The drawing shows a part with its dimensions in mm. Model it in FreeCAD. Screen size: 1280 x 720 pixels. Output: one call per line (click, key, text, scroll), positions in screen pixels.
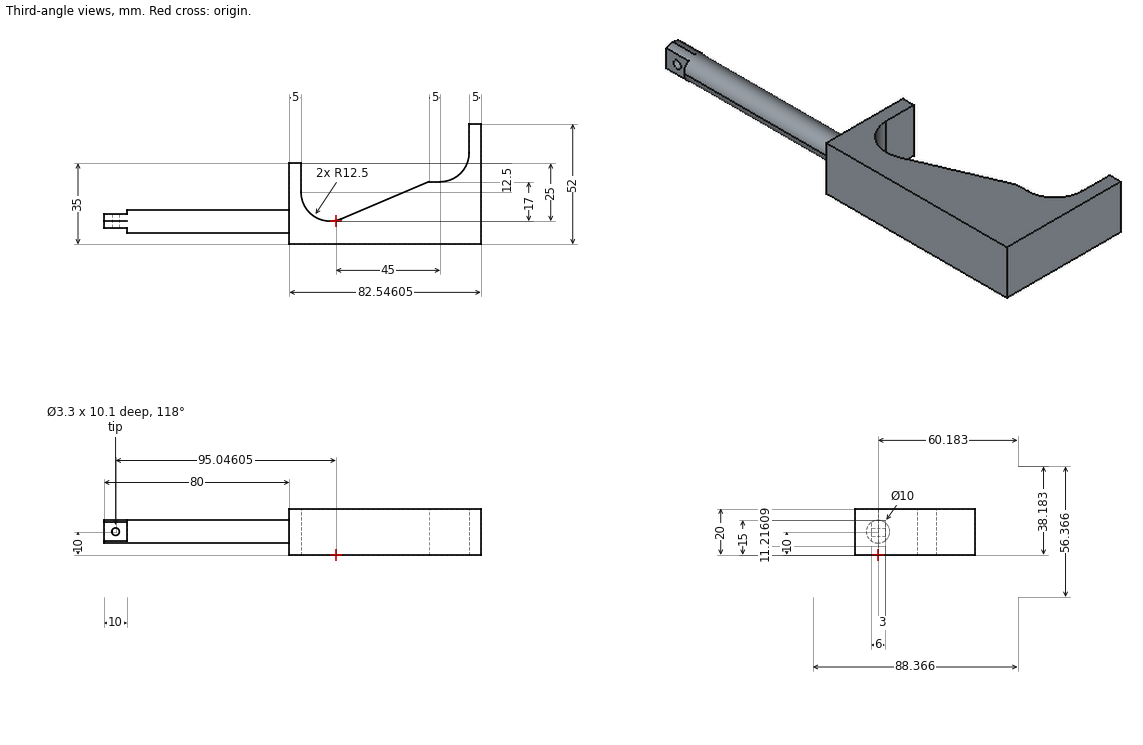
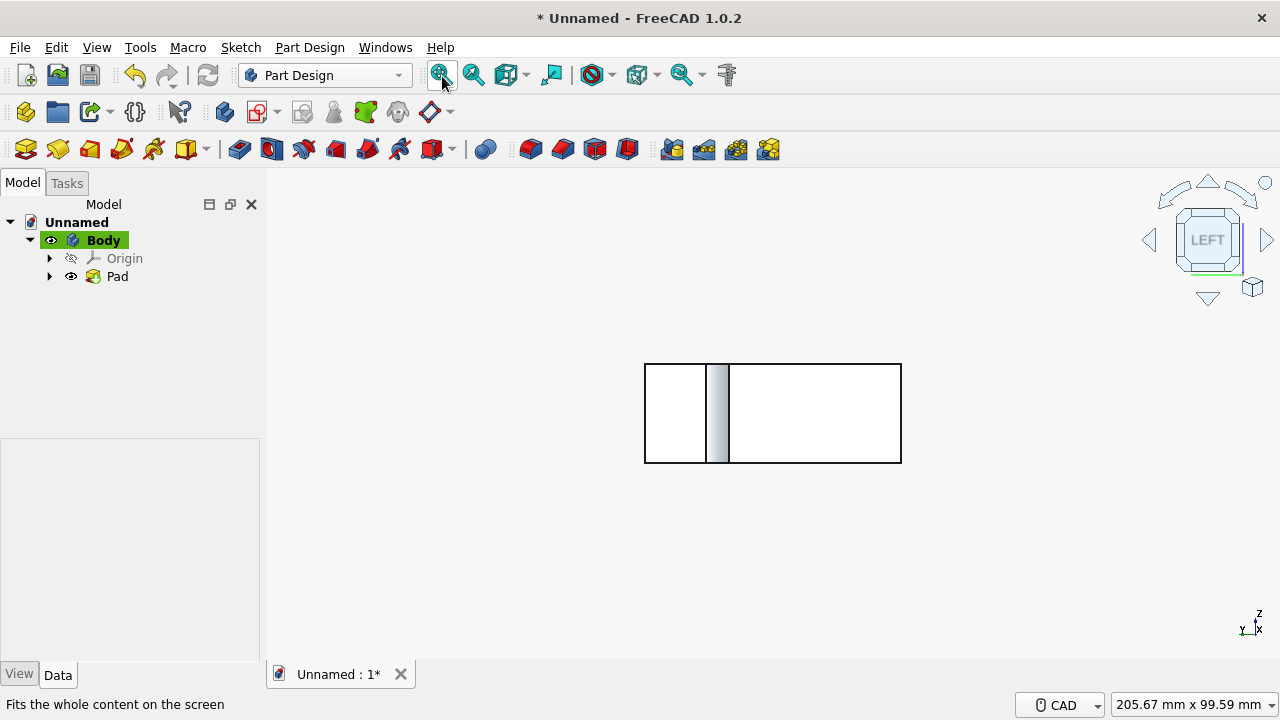
click(790, 412)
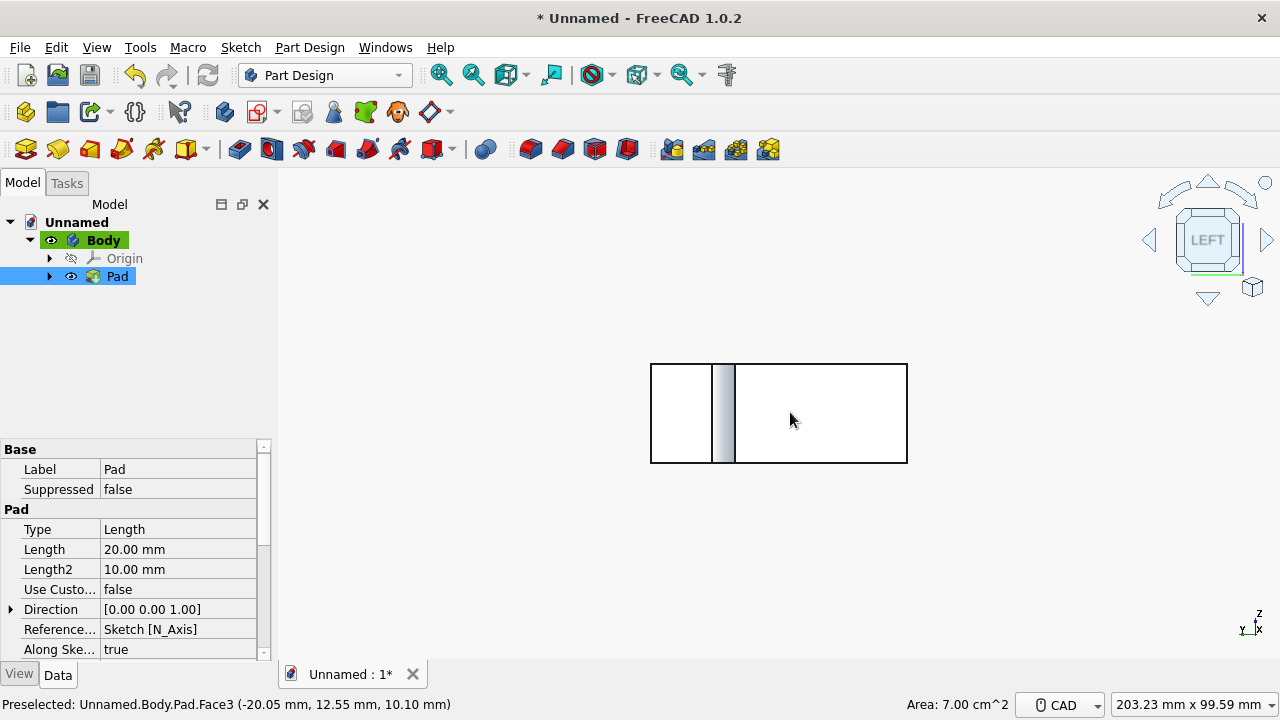
click(258, 112)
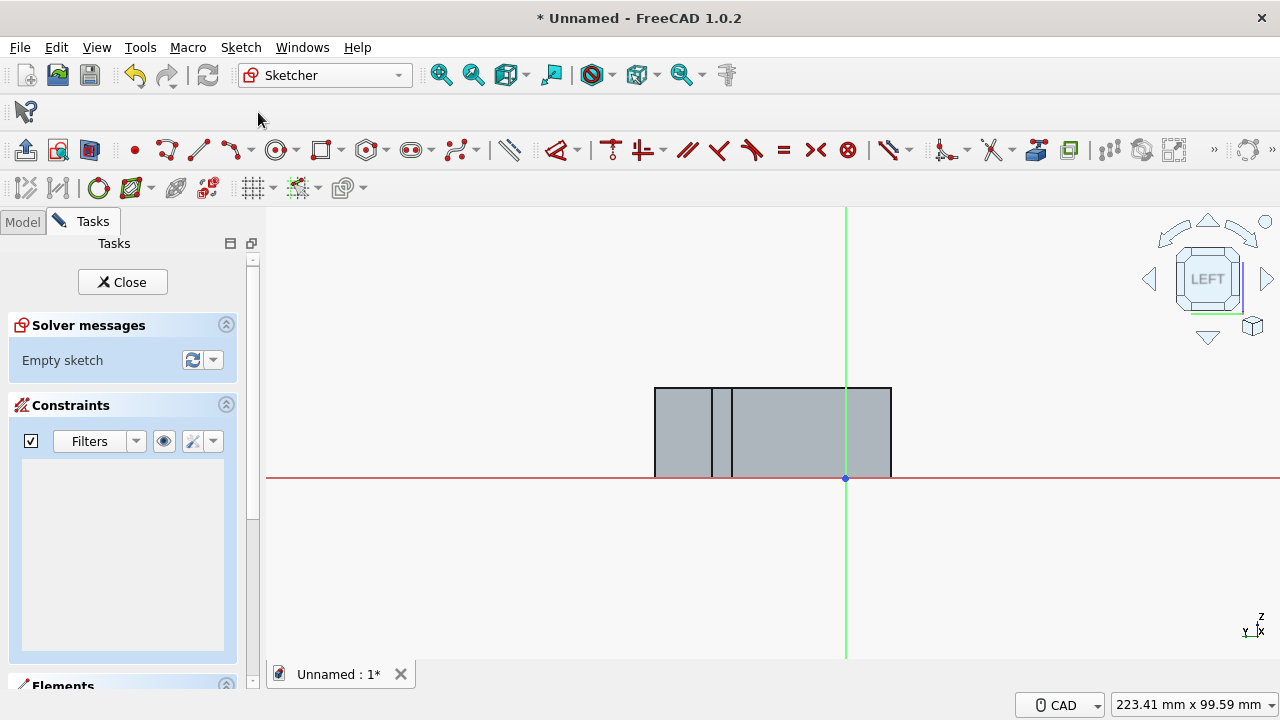
scroll(892, 448, up, 7)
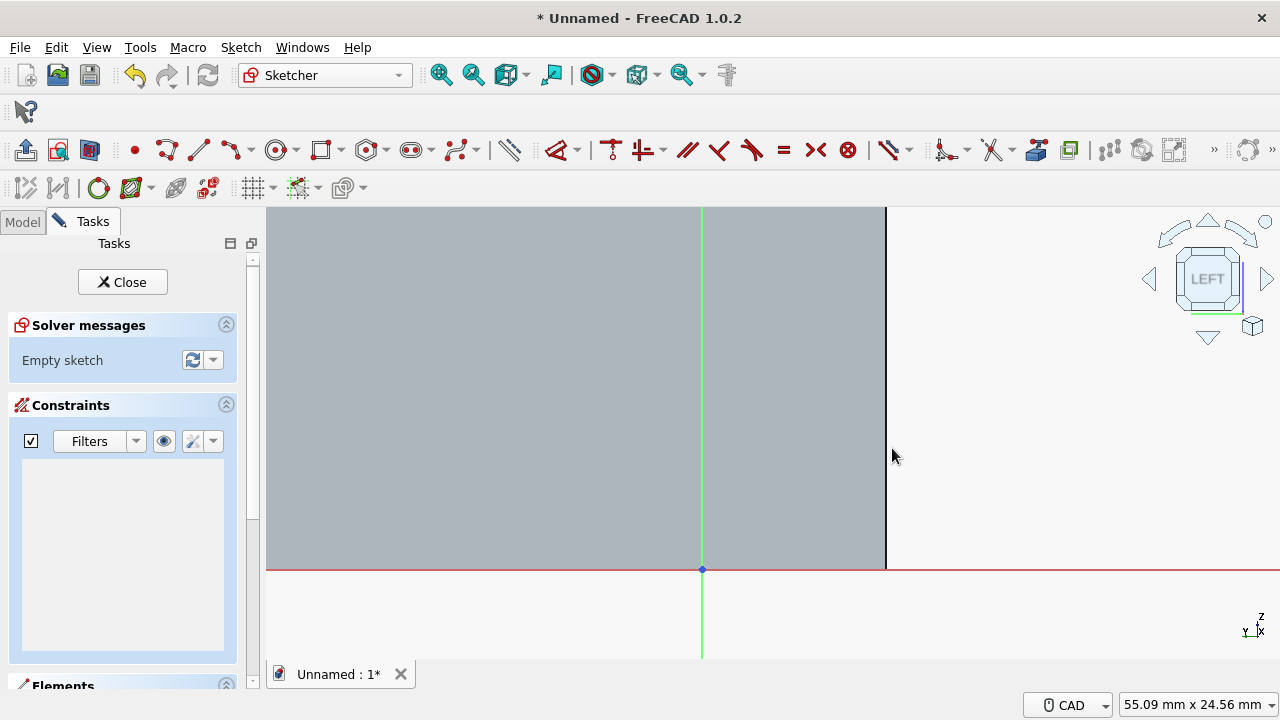
click(276, 150)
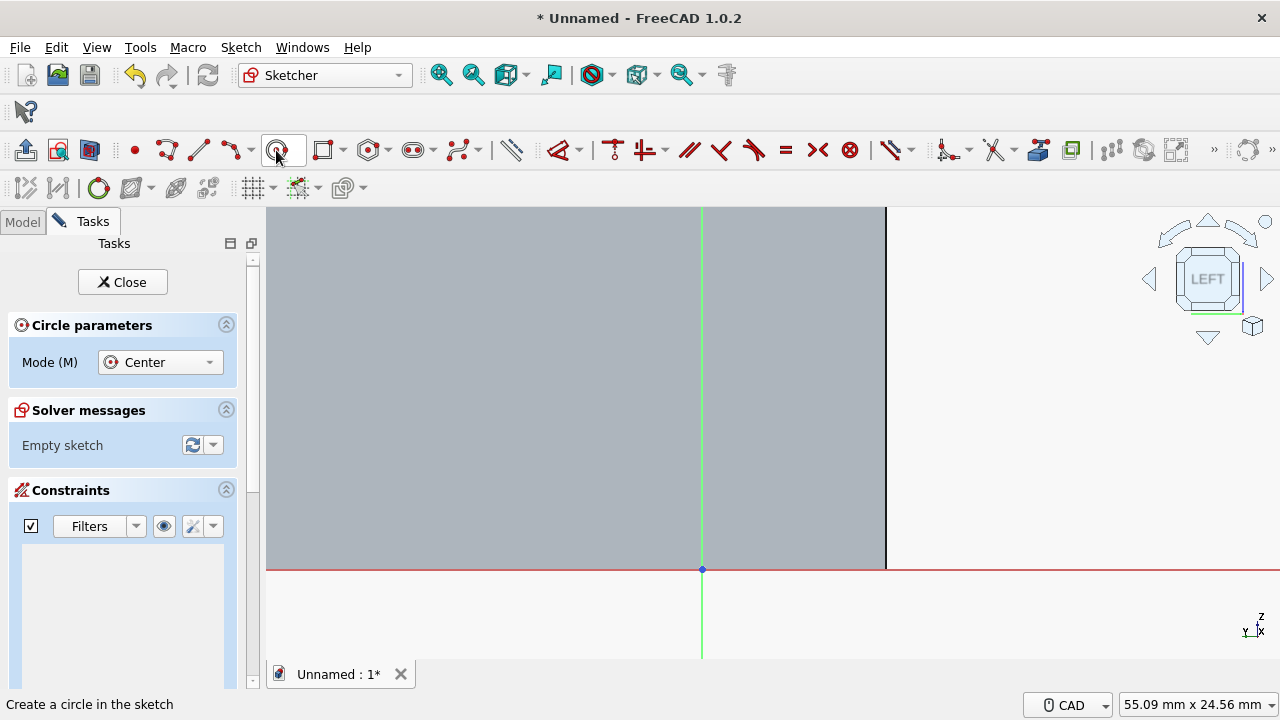
click(702, 386)
click(767, 320)
key(Escape)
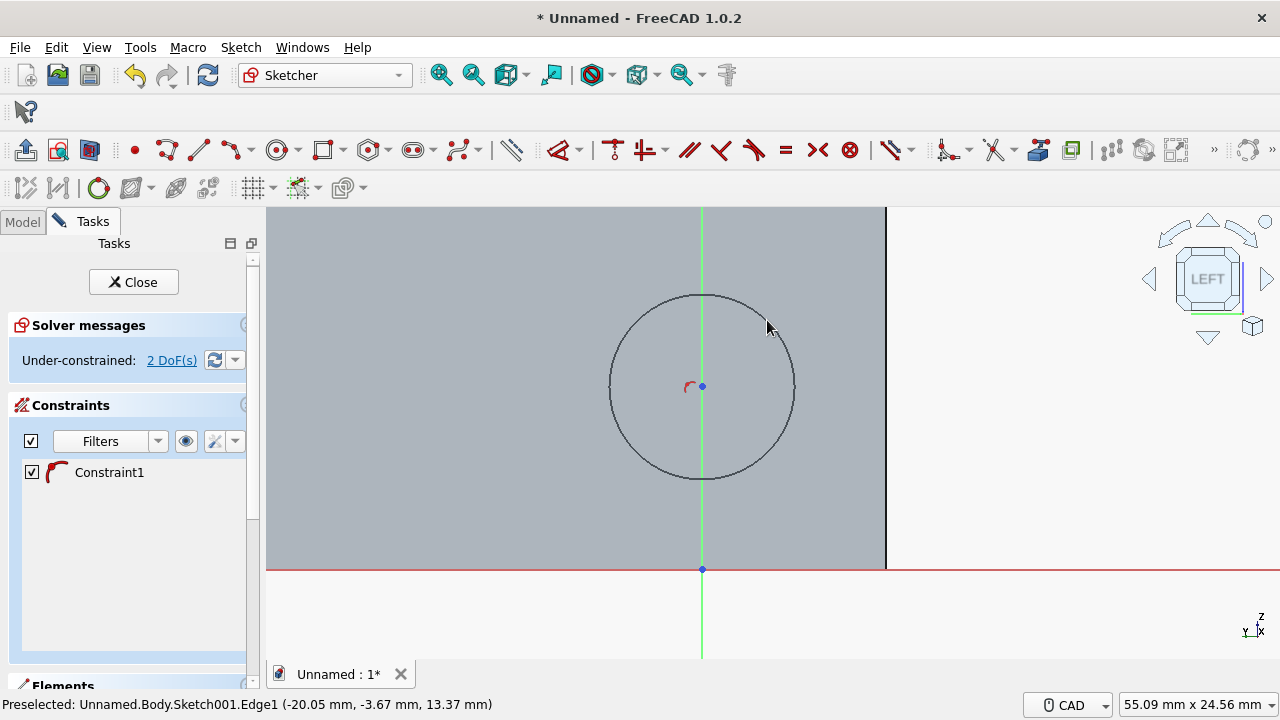
click(558, 150)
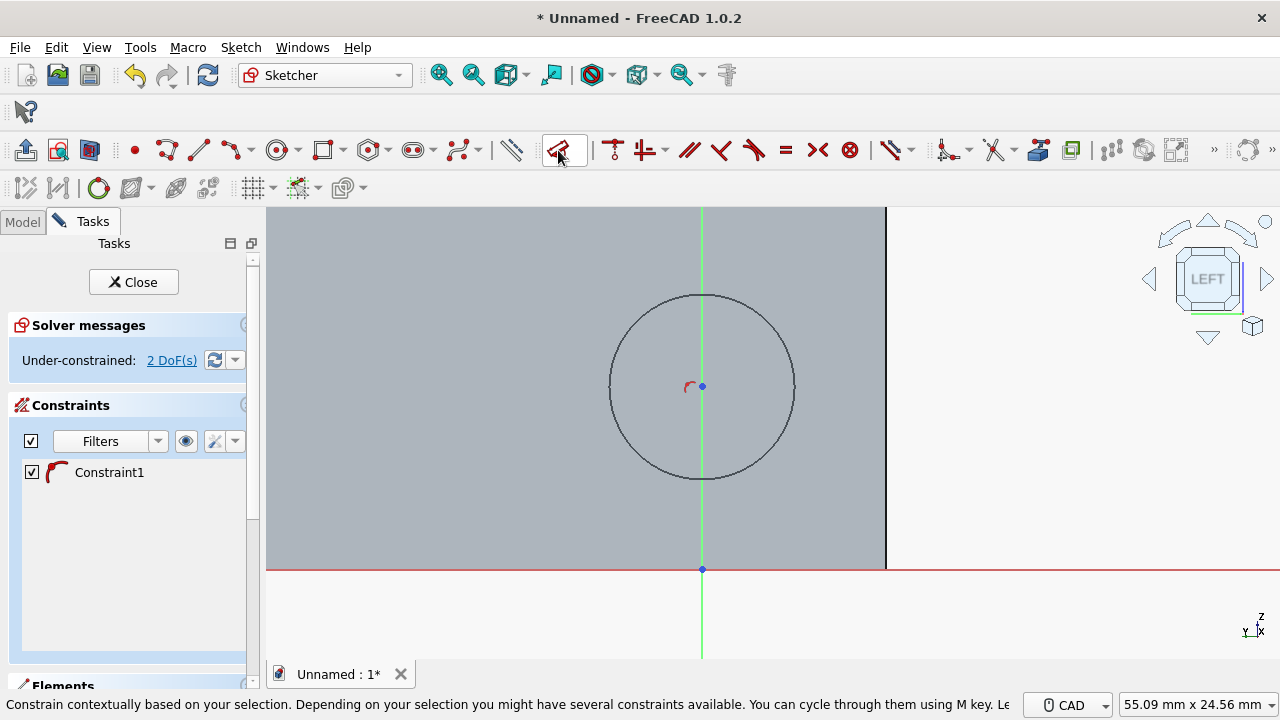
click(767, 321)
click(789, 298)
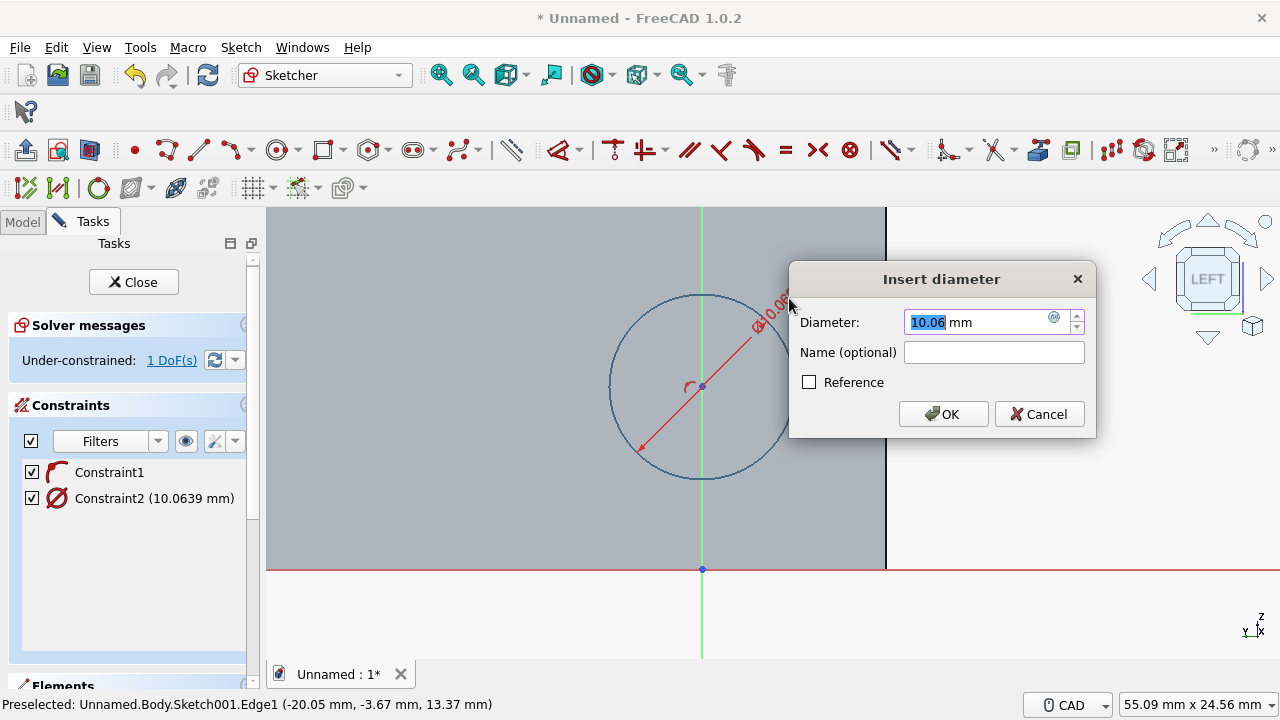
text(10)
key(Return)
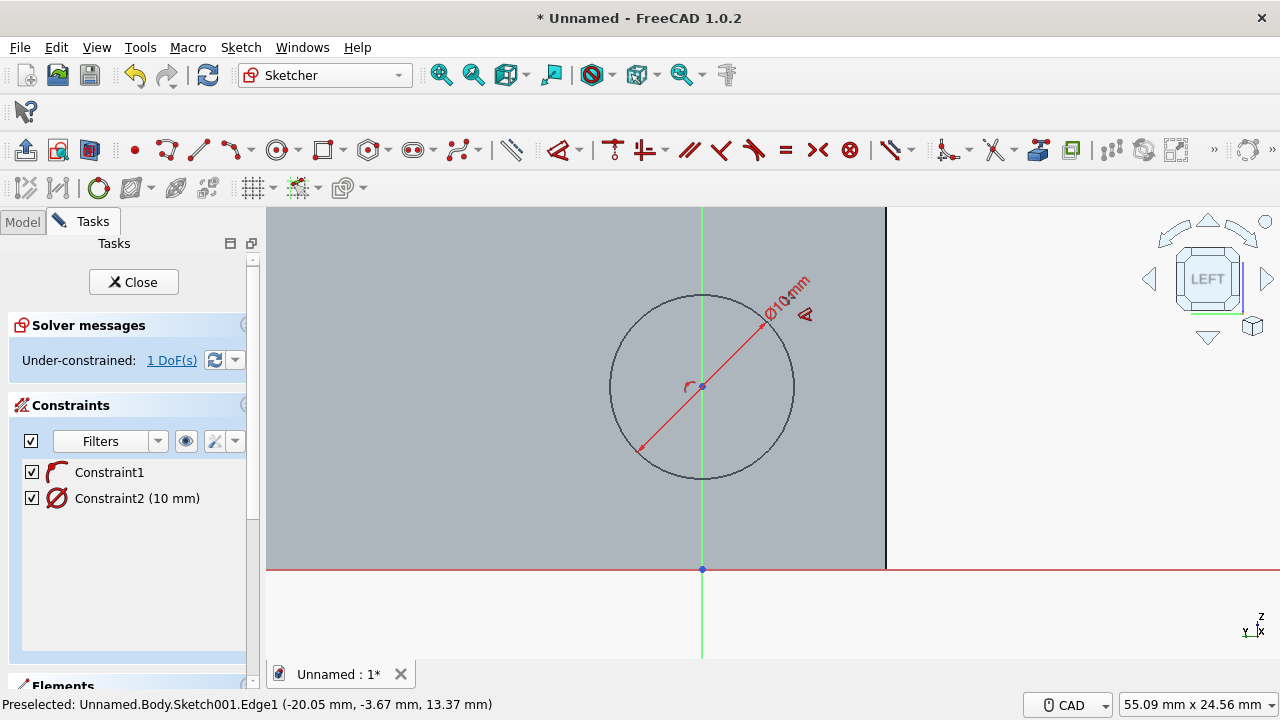
click(702, 387)
click(736, 436)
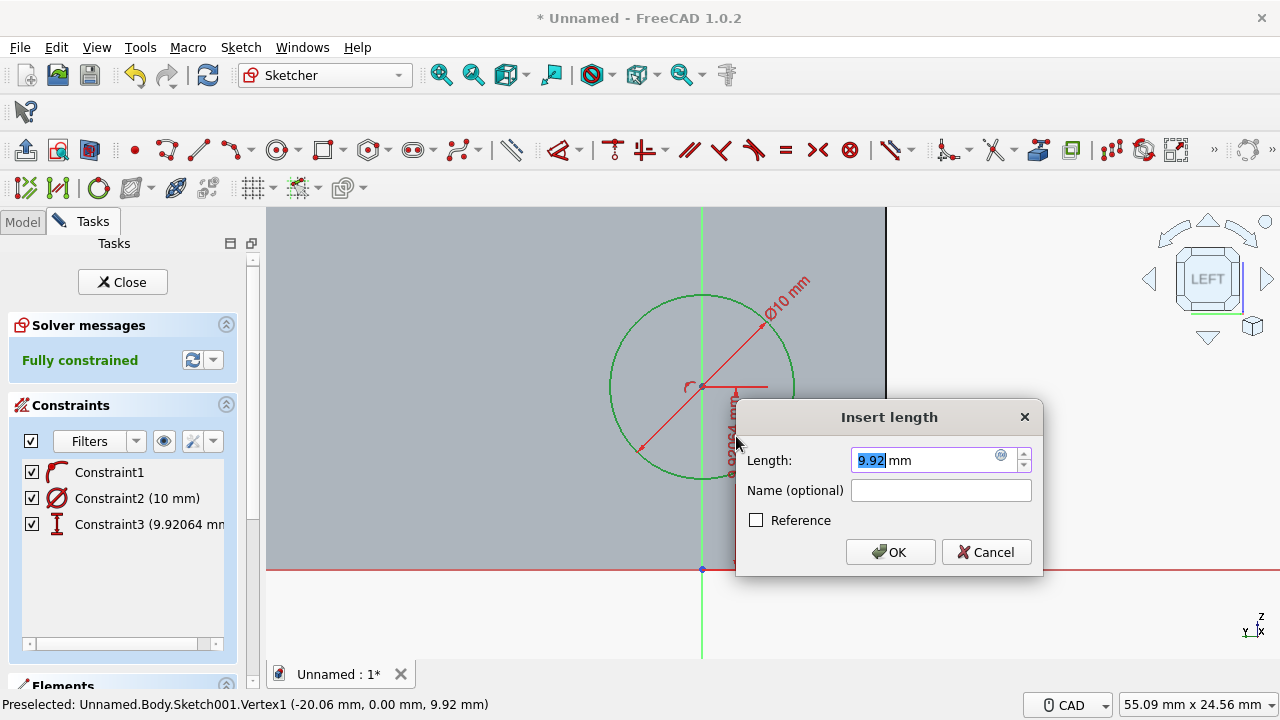
text(10)
key(Return)
key(Escape)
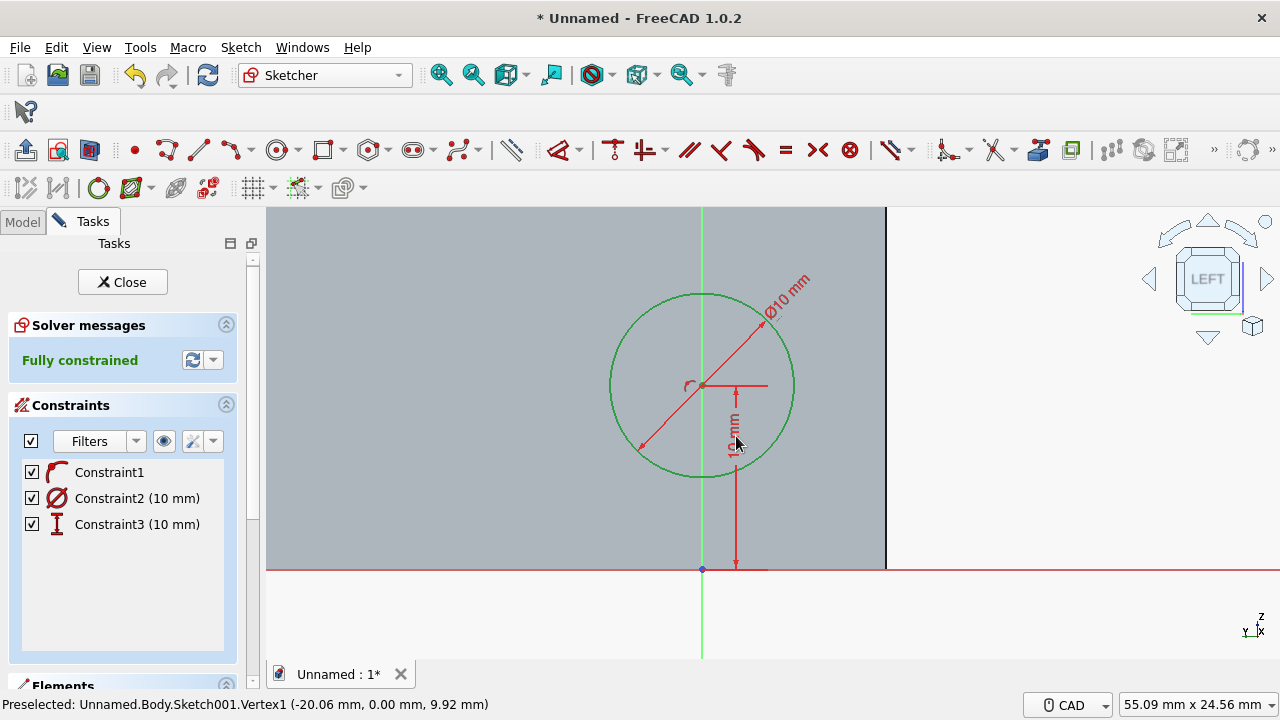
click(123, 282)